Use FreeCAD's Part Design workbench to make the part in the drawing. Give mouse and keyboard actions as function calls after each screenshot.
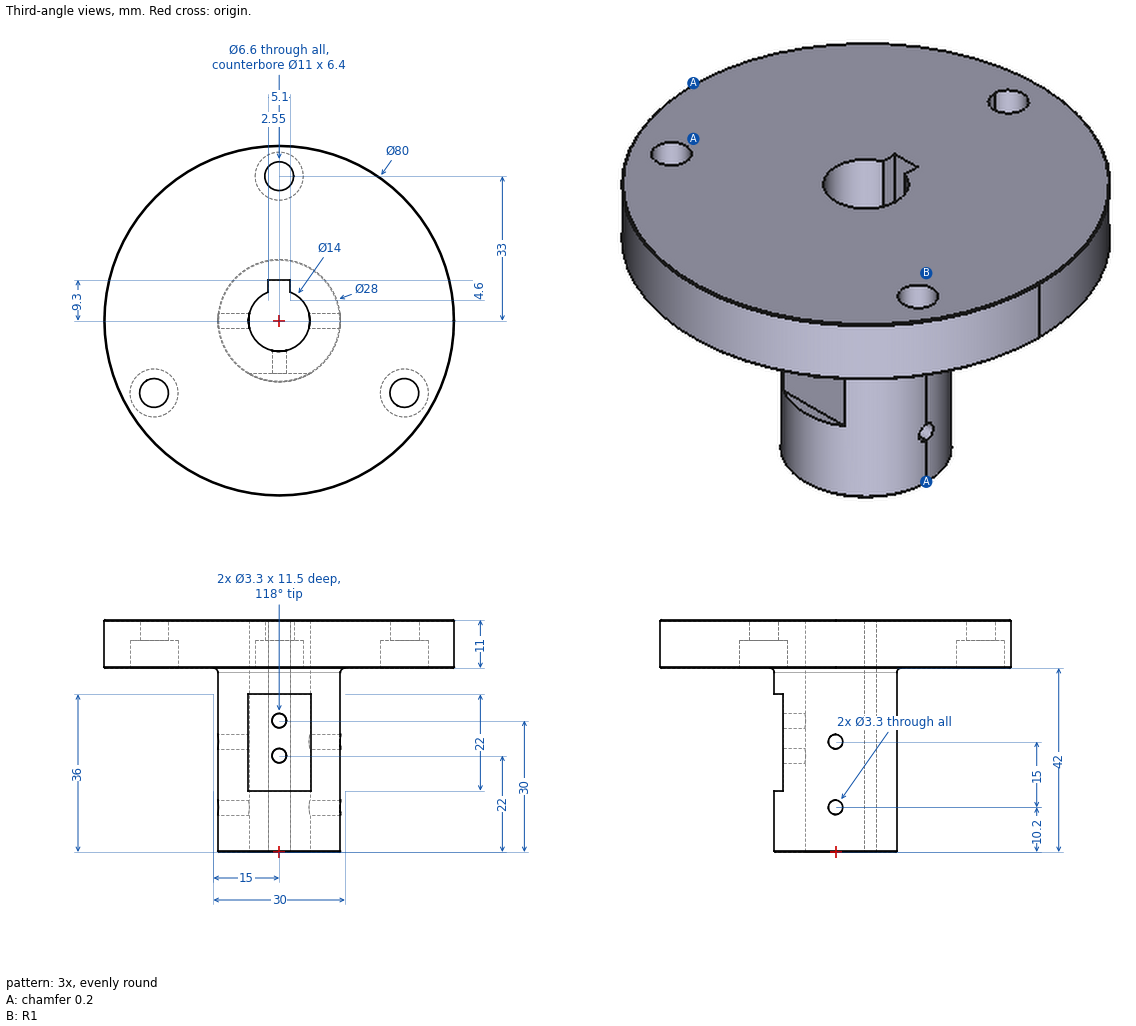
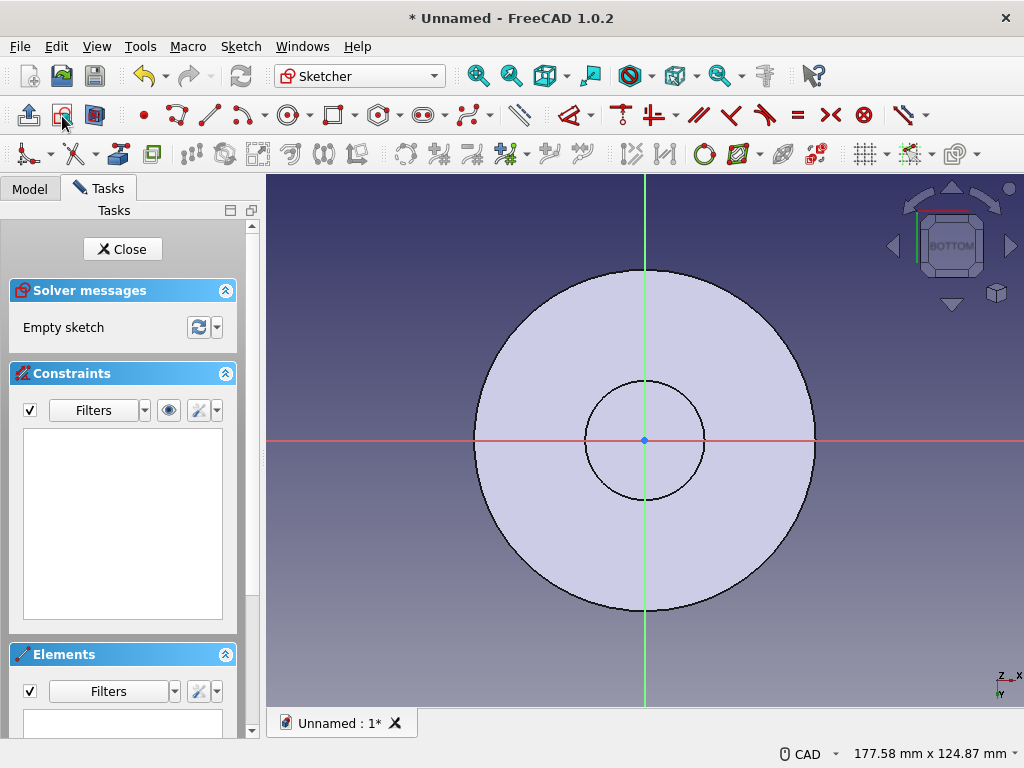
scroll(658, 440, up, 9)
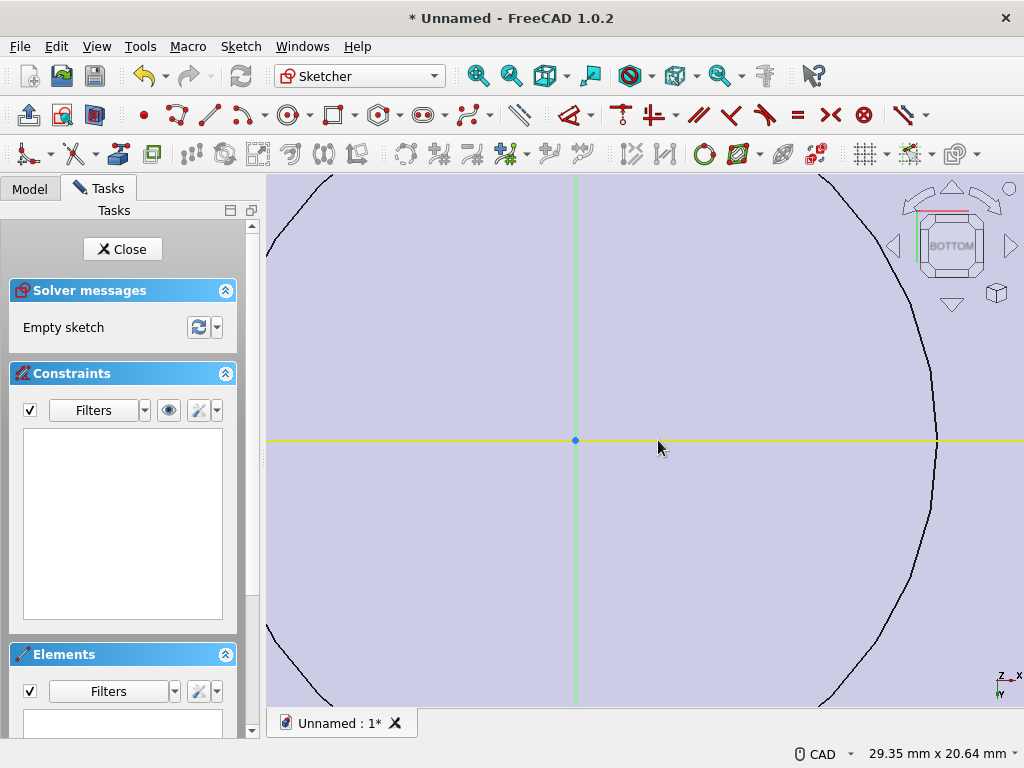
key(g)
key(c)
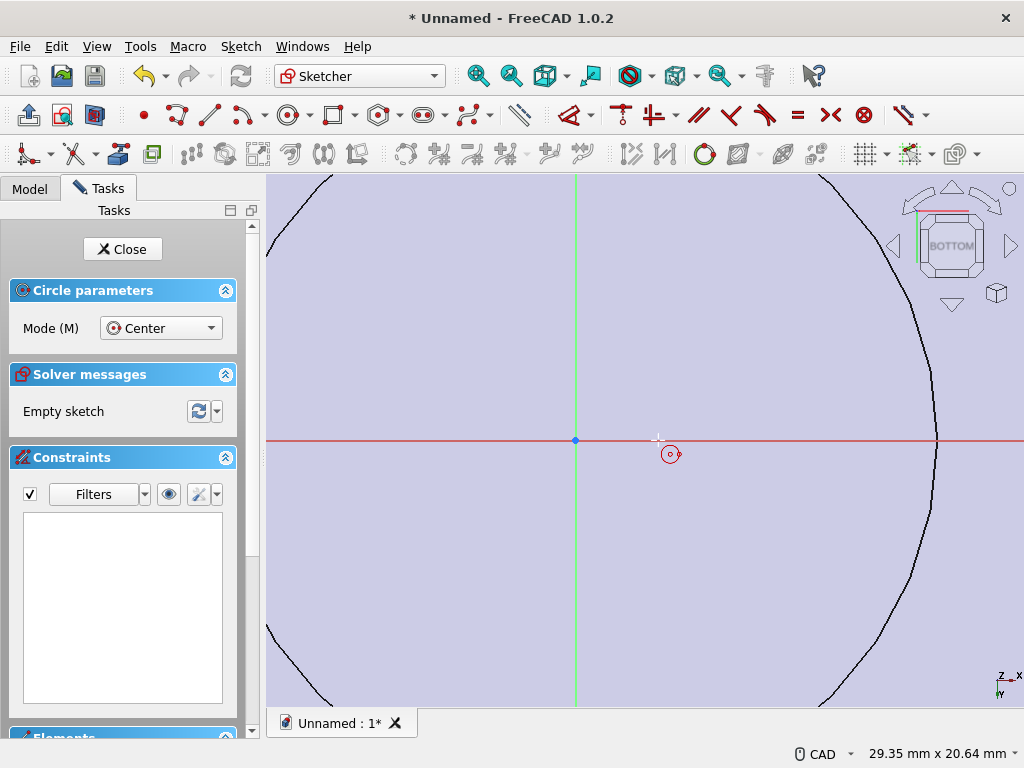
click(576, 440)
move(704, 313)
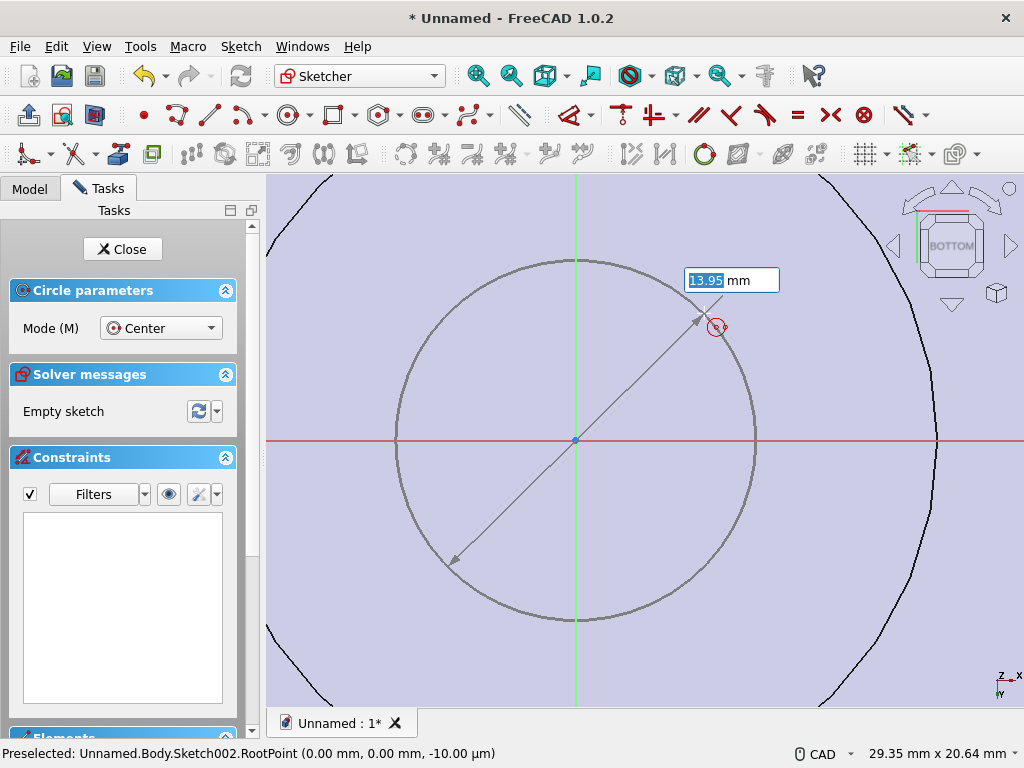
text(14)
key(Return)
key(Escape)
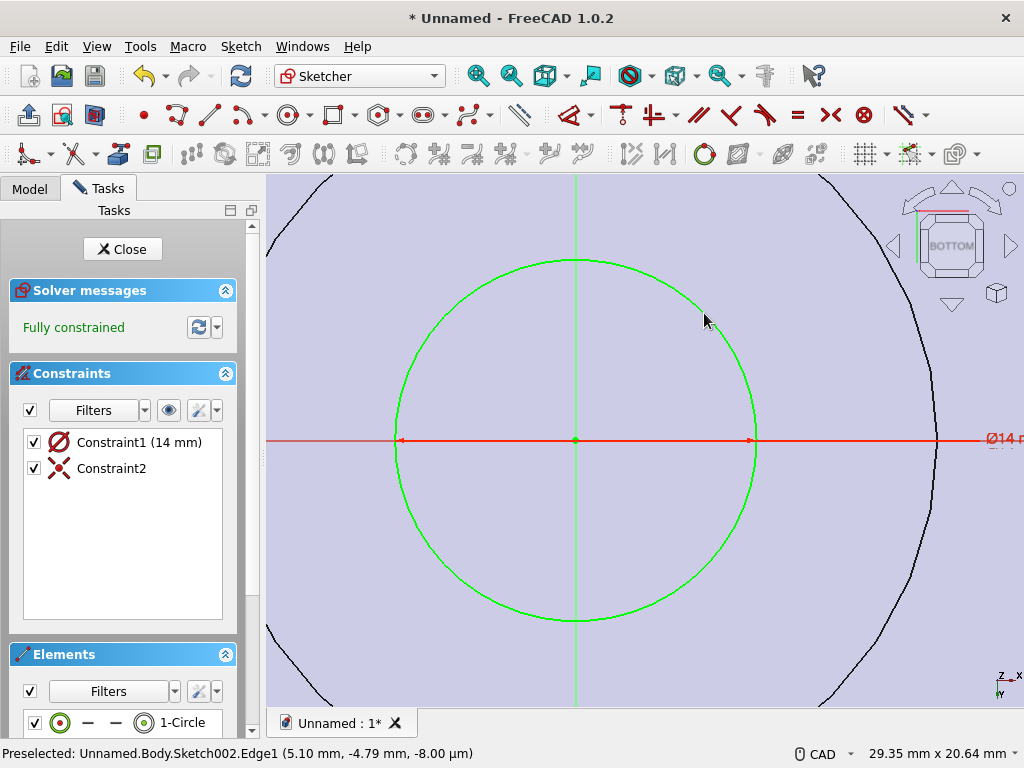
click(123, 249)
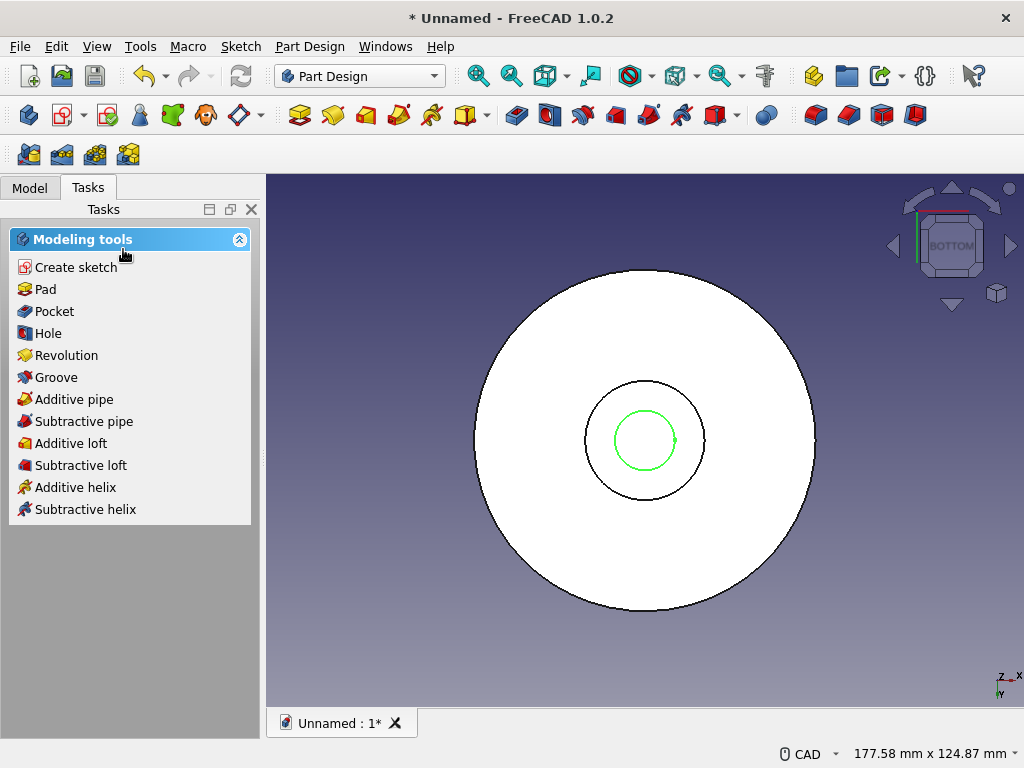
click(517, 116)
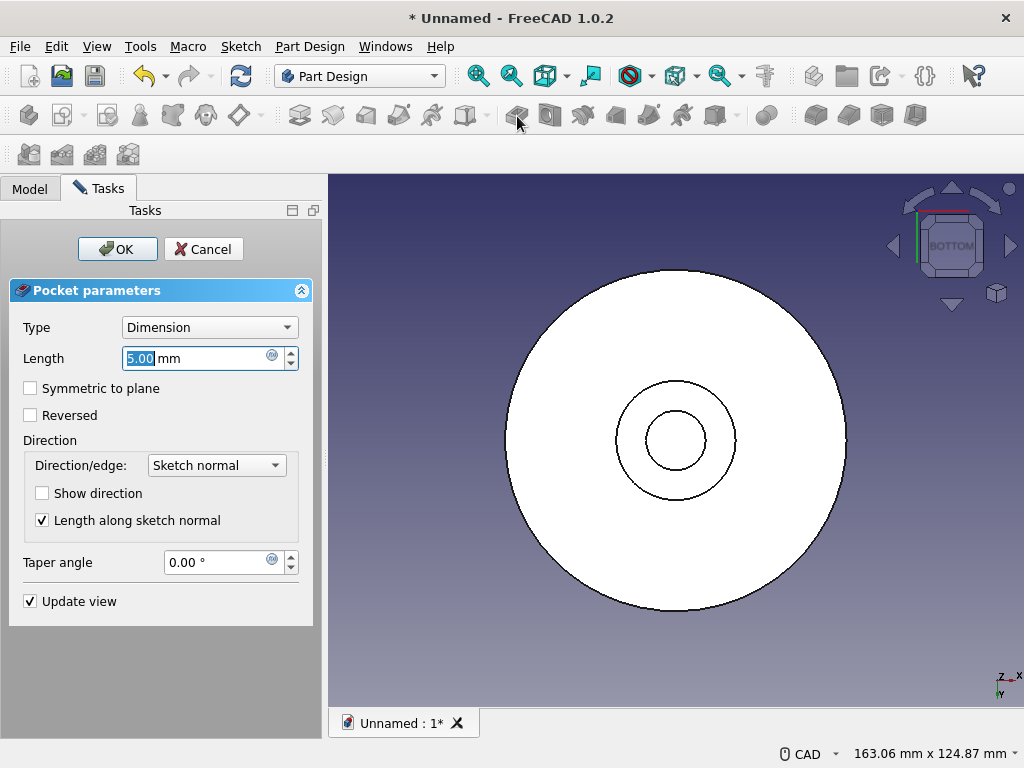
click(210, 328)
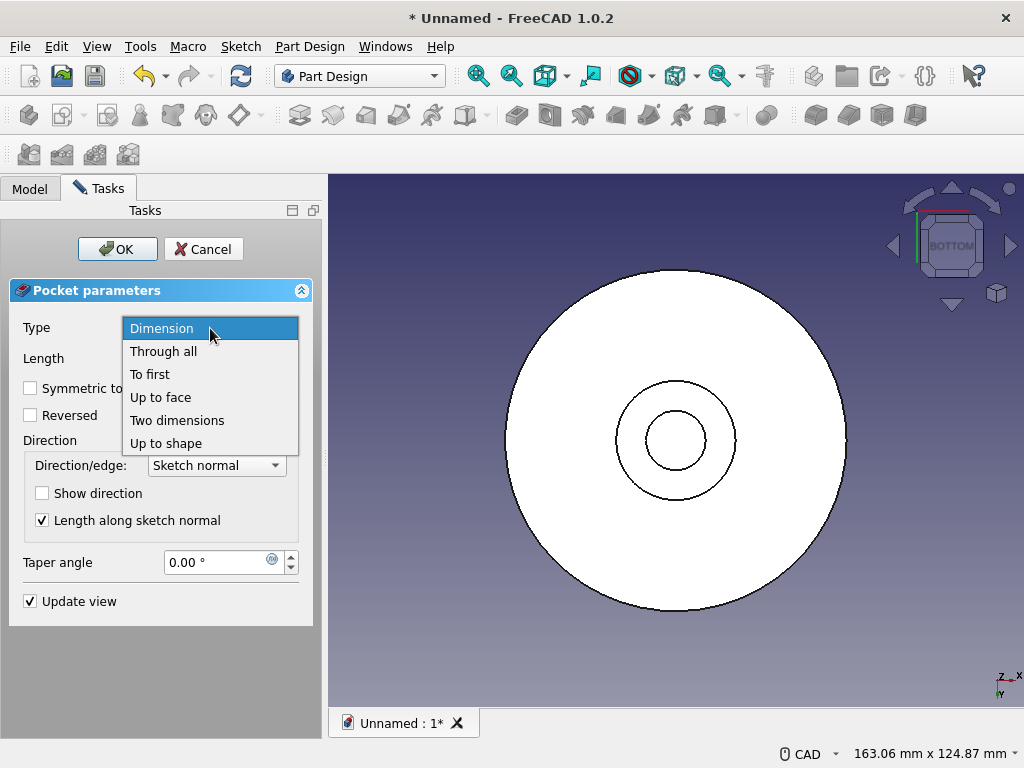
click(208, 352)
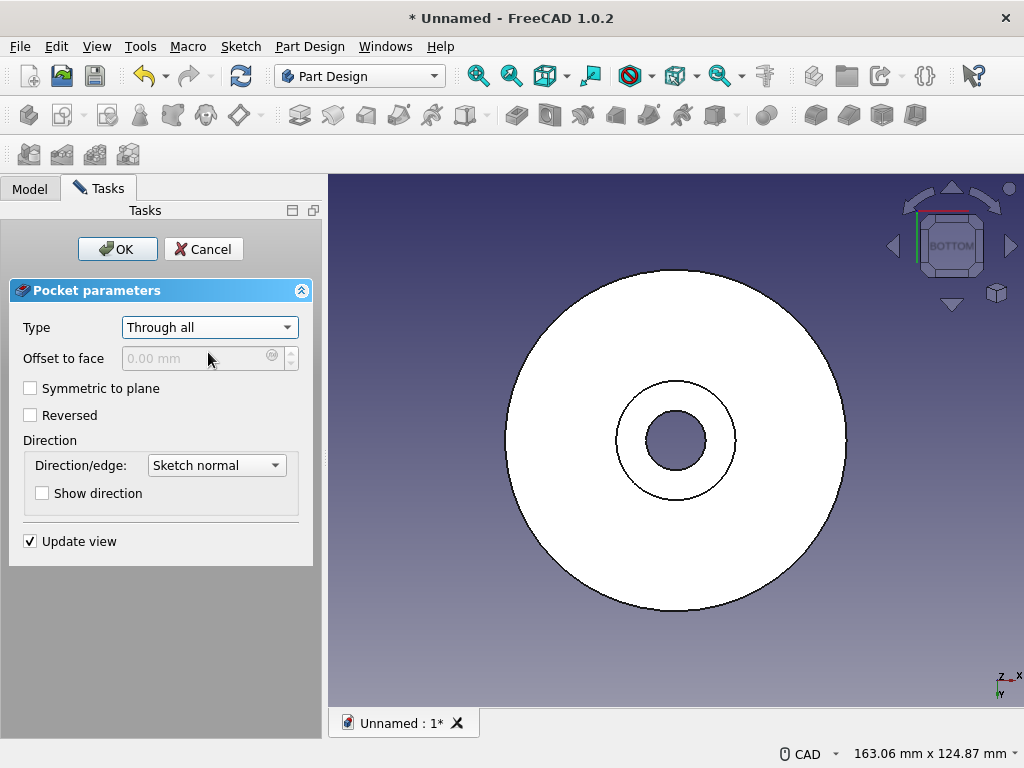
click(118, 249)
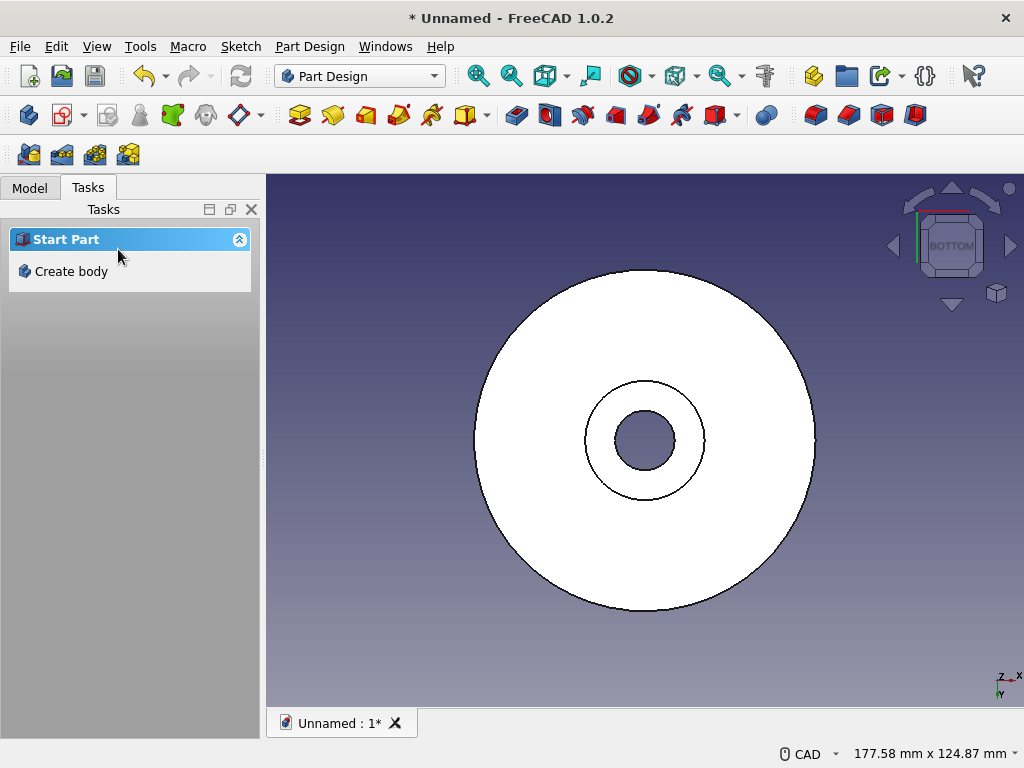
click(547, 488)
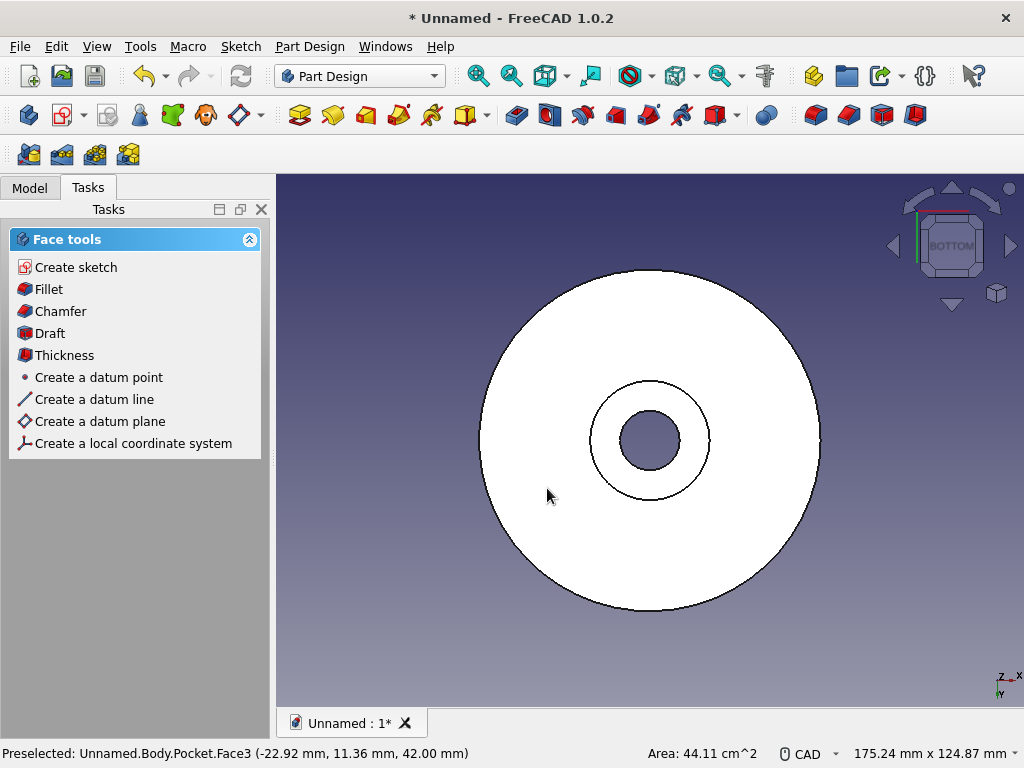
click(62, 116)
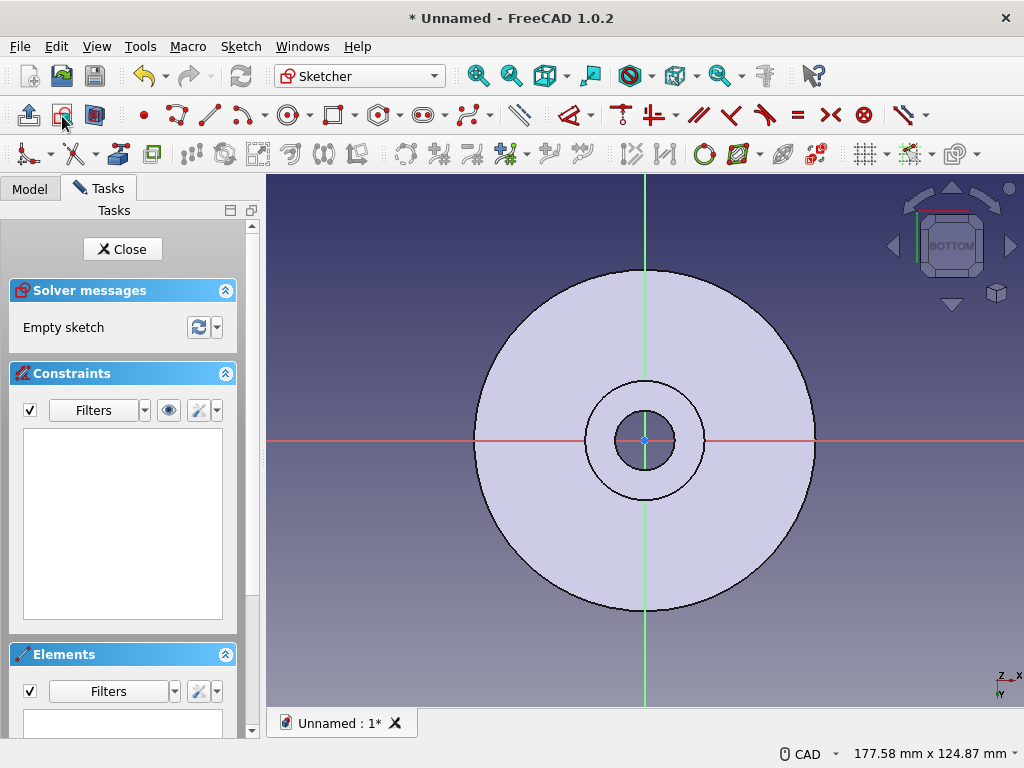
key(q)
key(s)